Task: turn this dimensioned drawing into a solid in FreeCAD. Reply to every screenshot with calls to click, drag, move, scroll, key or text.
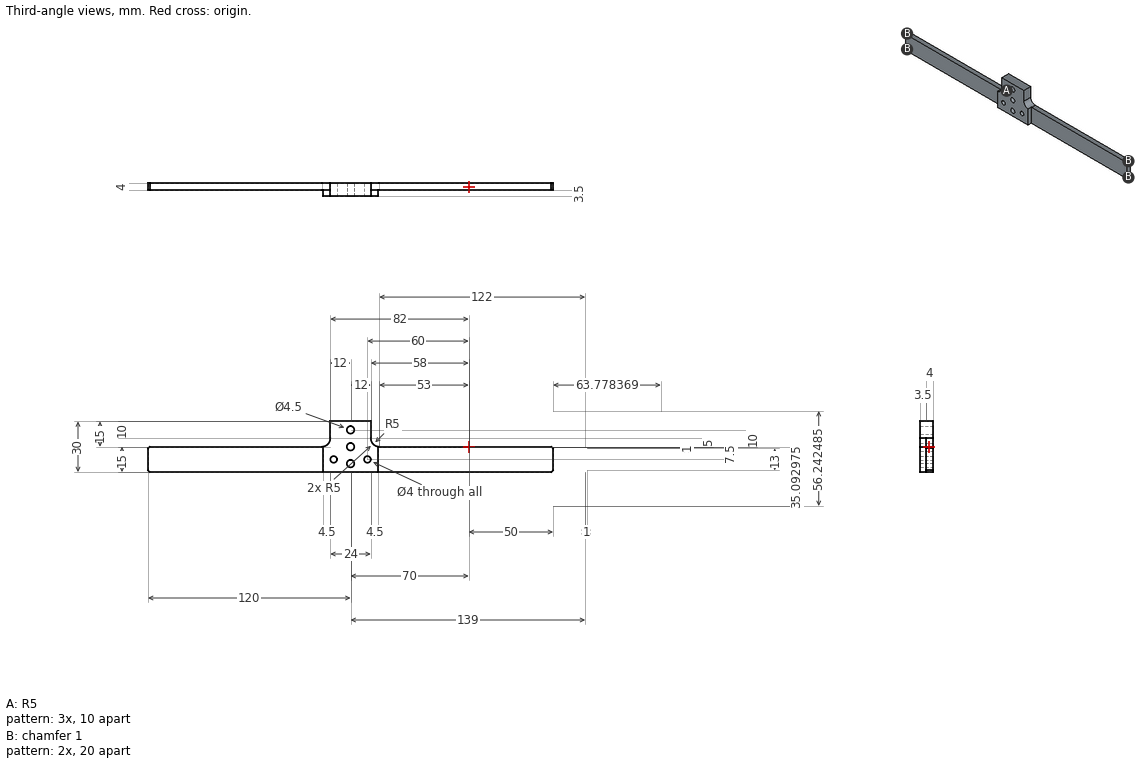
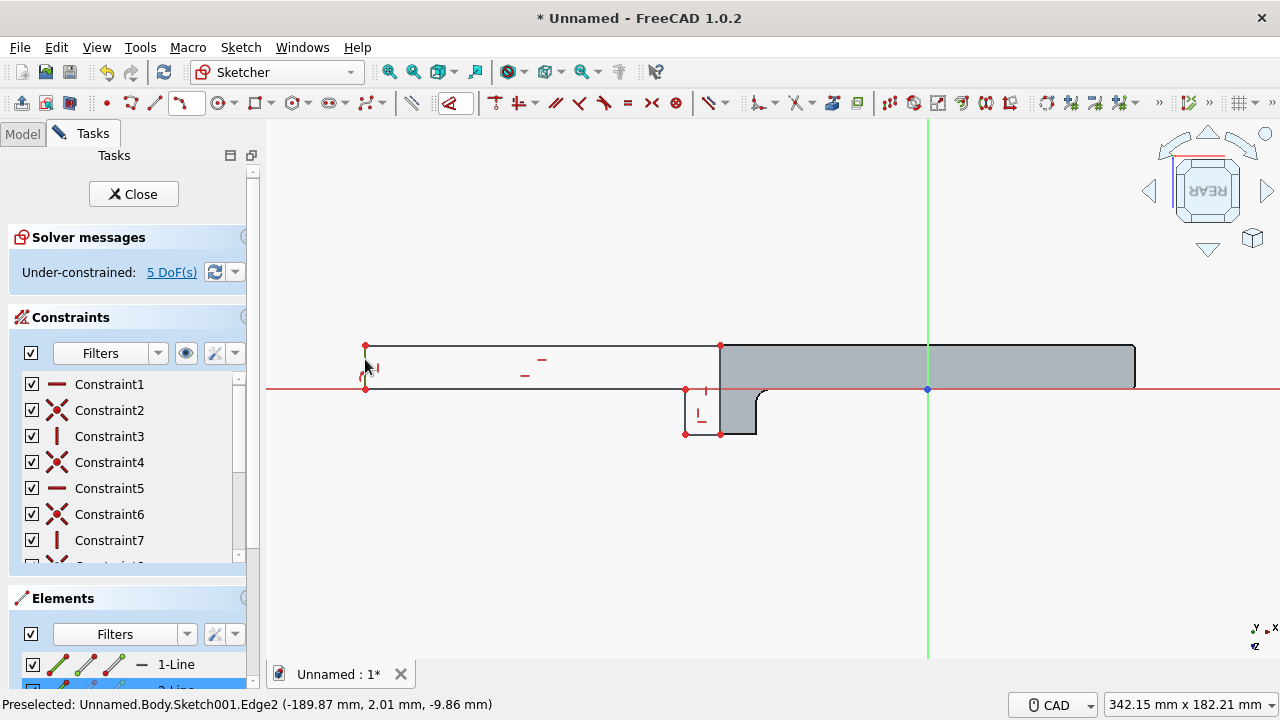
click(468, 104)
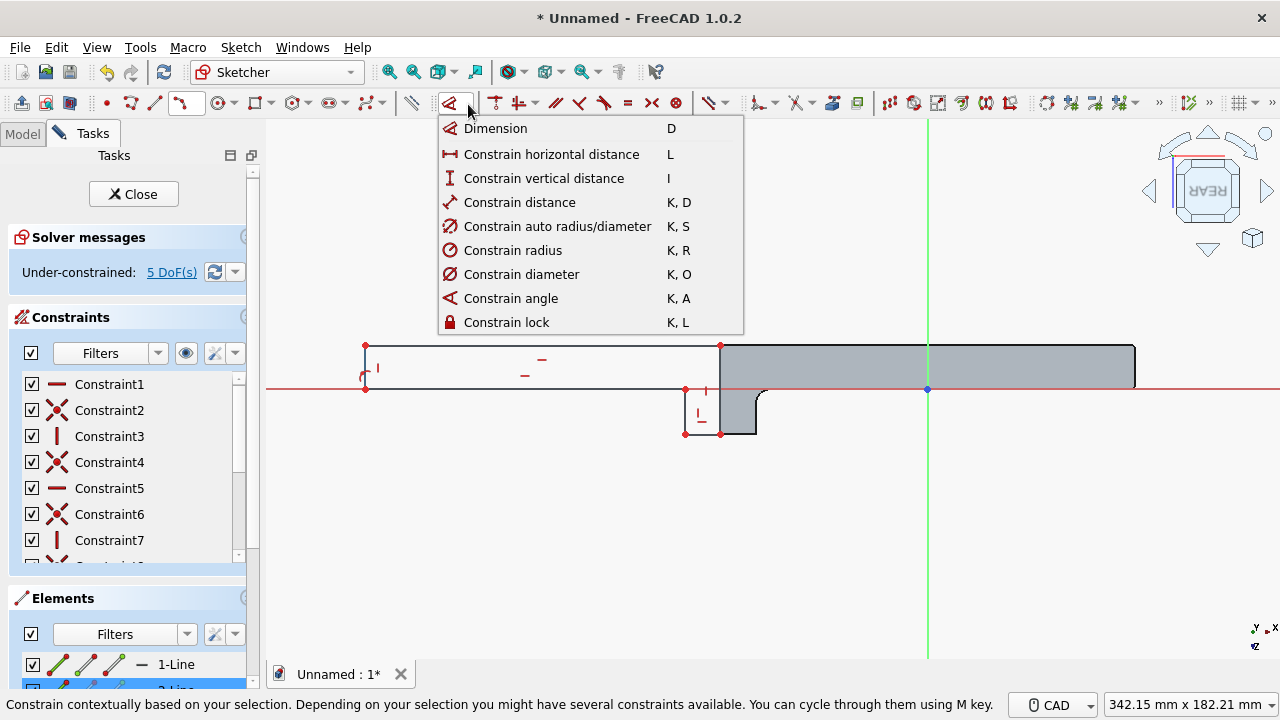
click(591, 178)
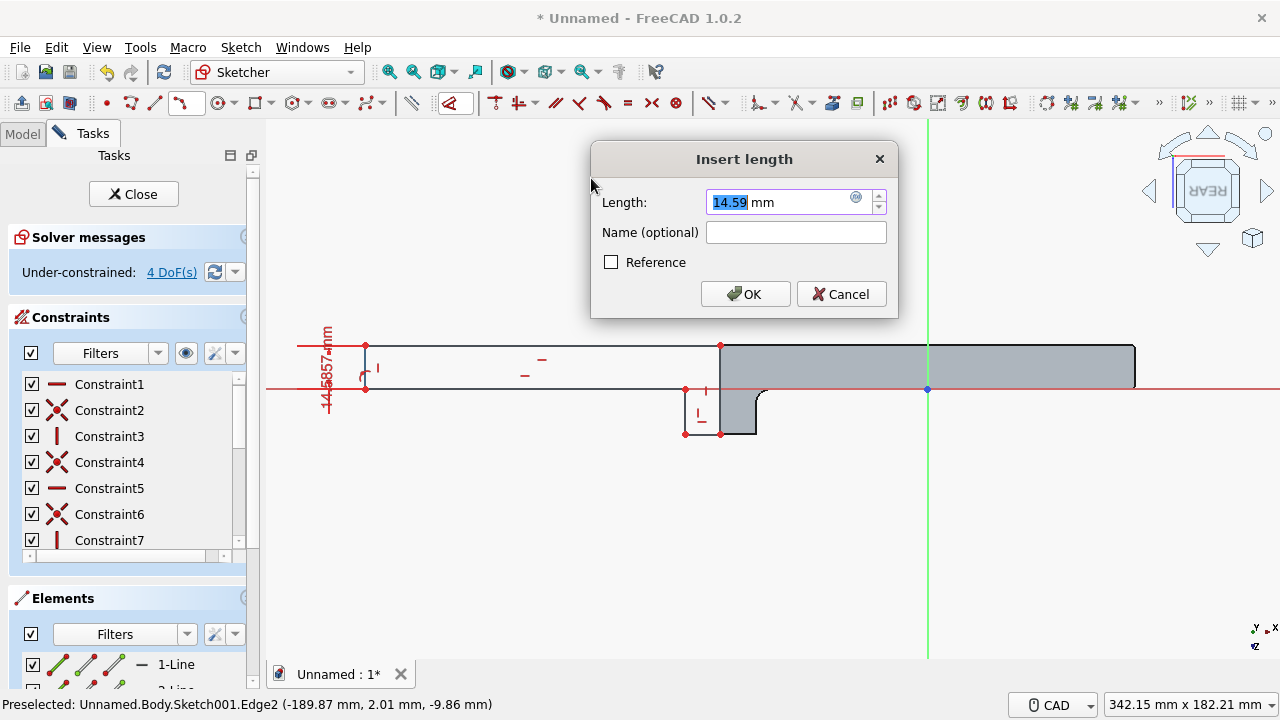
text(15)
key(Return)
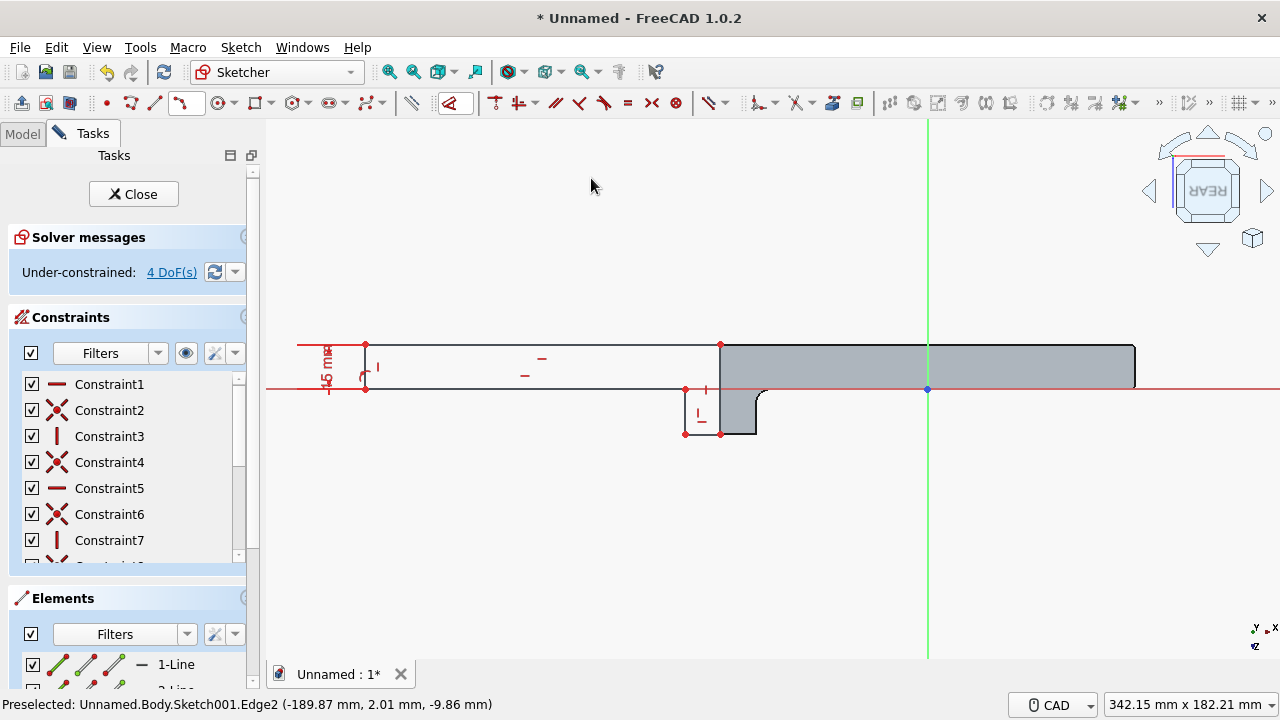
click(685, 403)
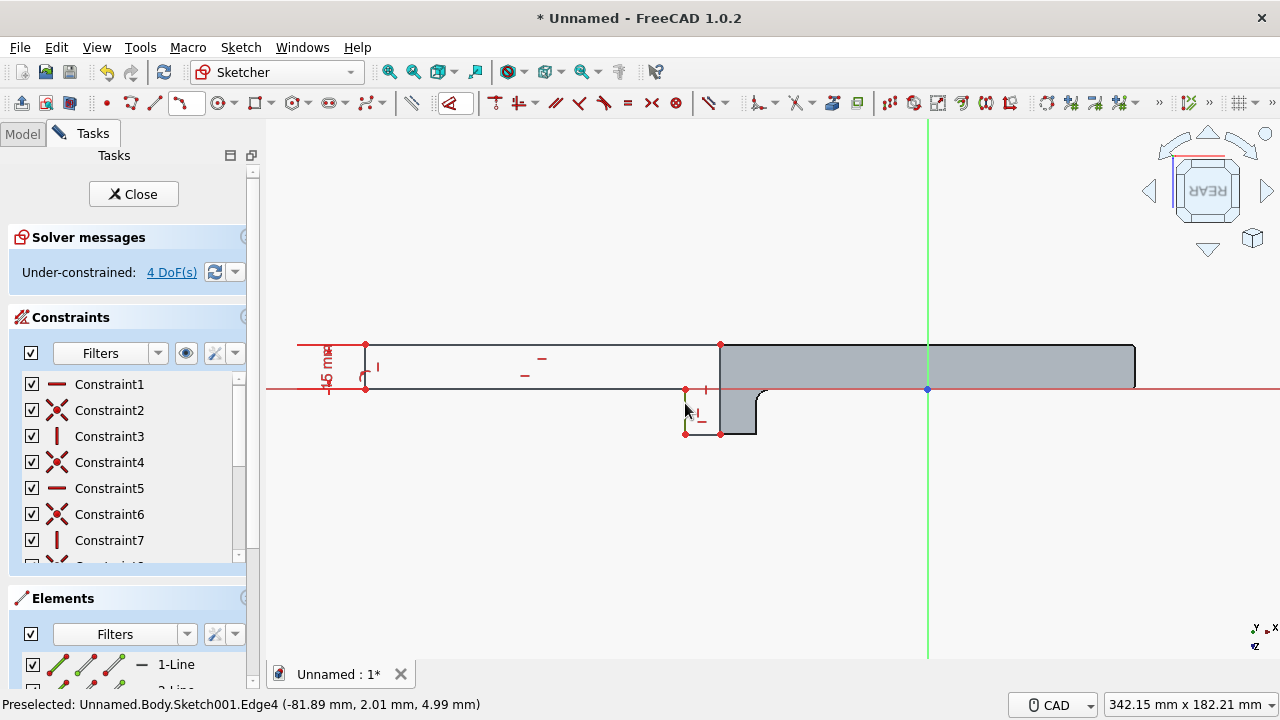
click(468, 104)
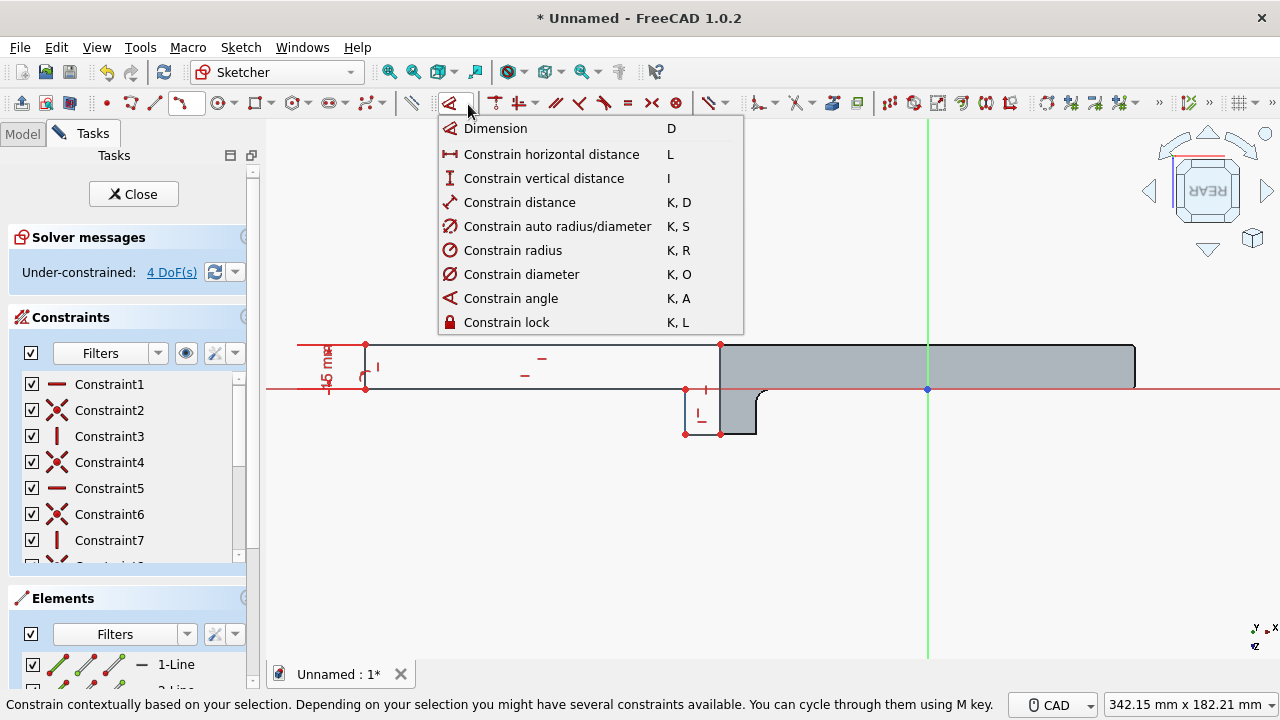
click(591, 178)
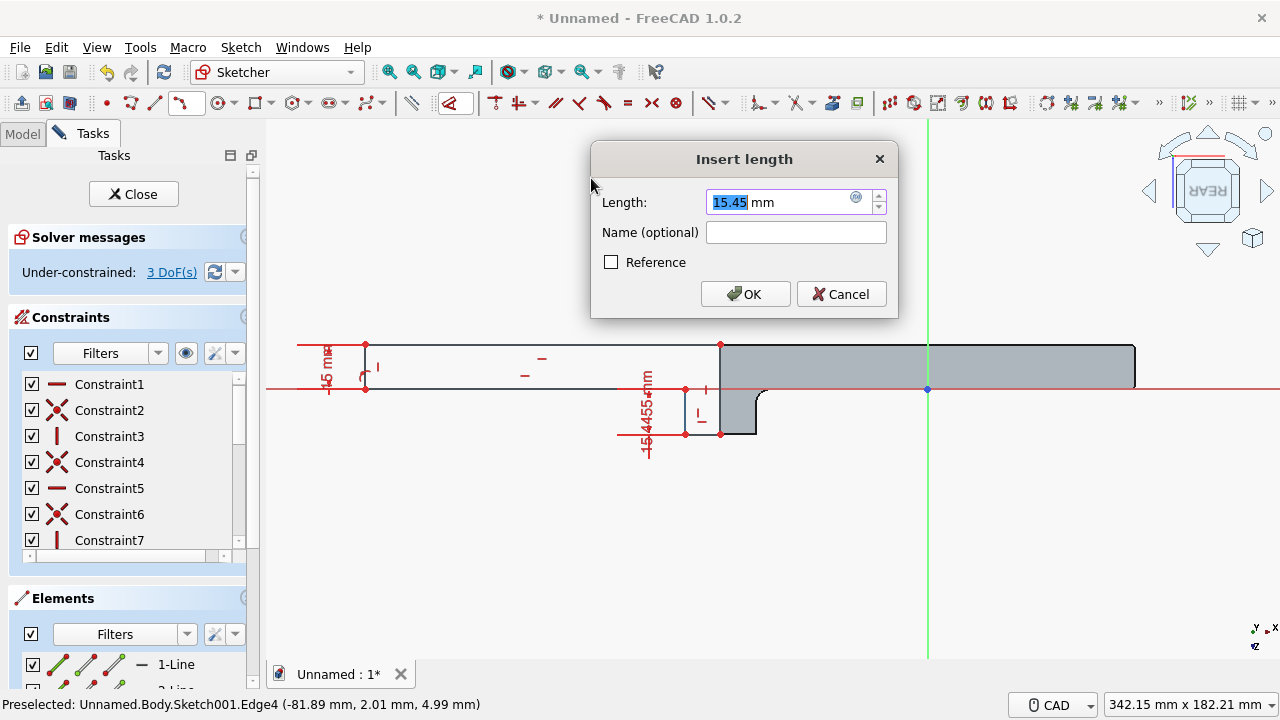
text(15)
key(Return)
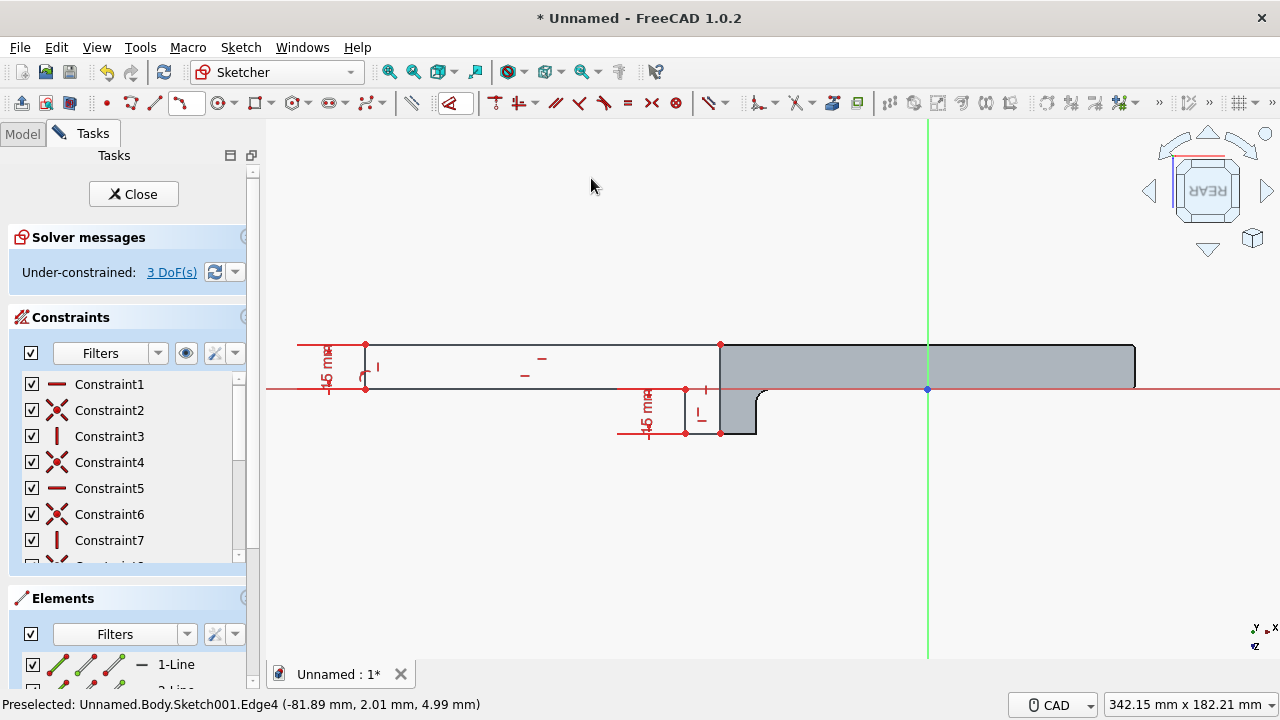
scroll(695, 434, up, 2)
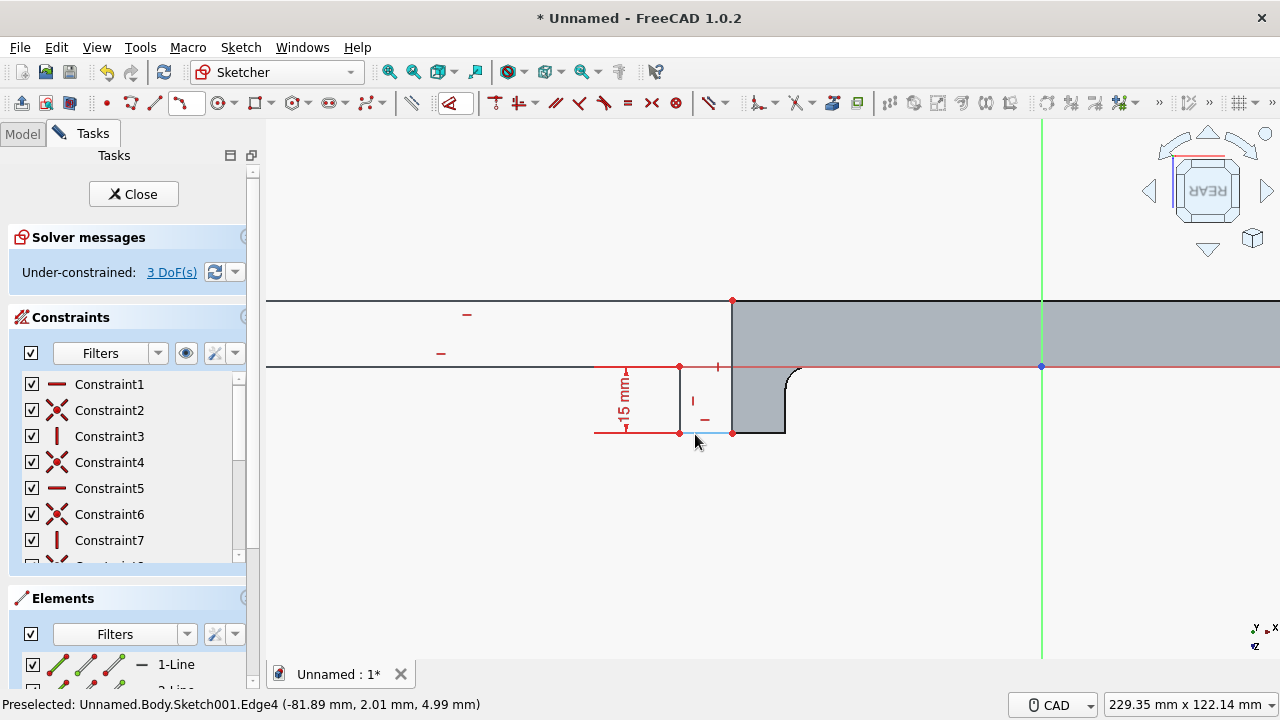
click(696, 433)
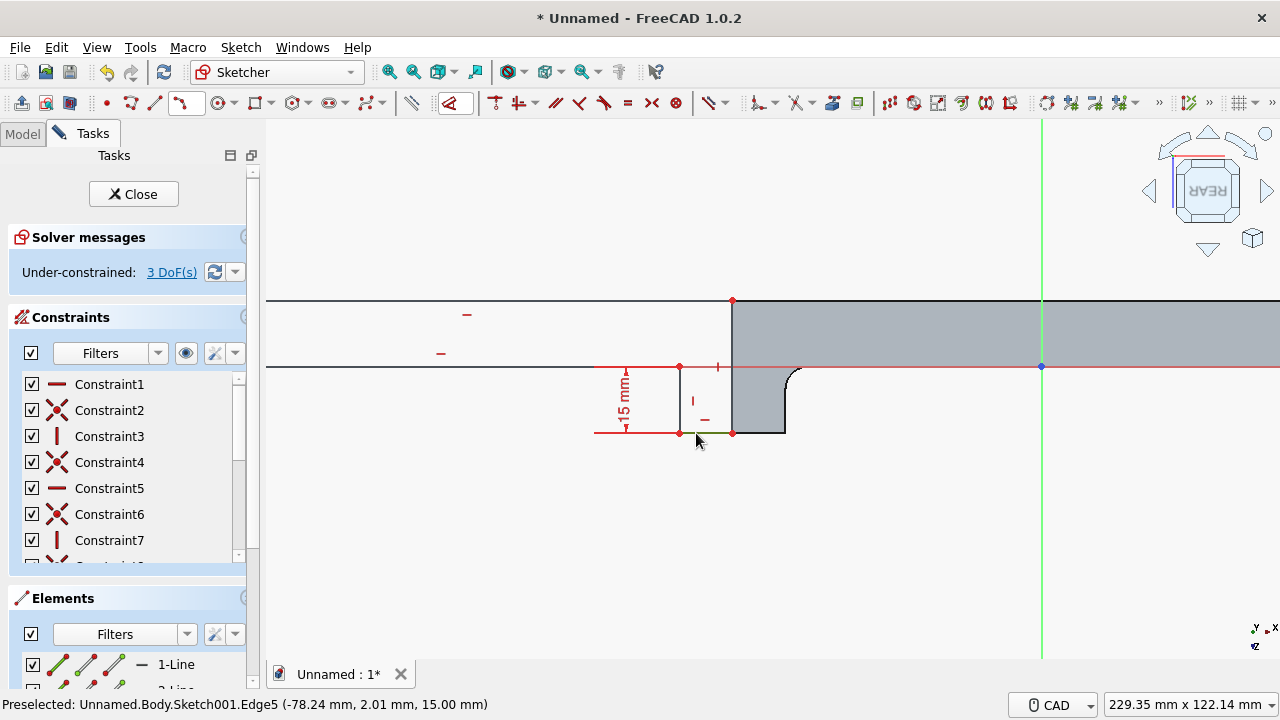
click(468, 104)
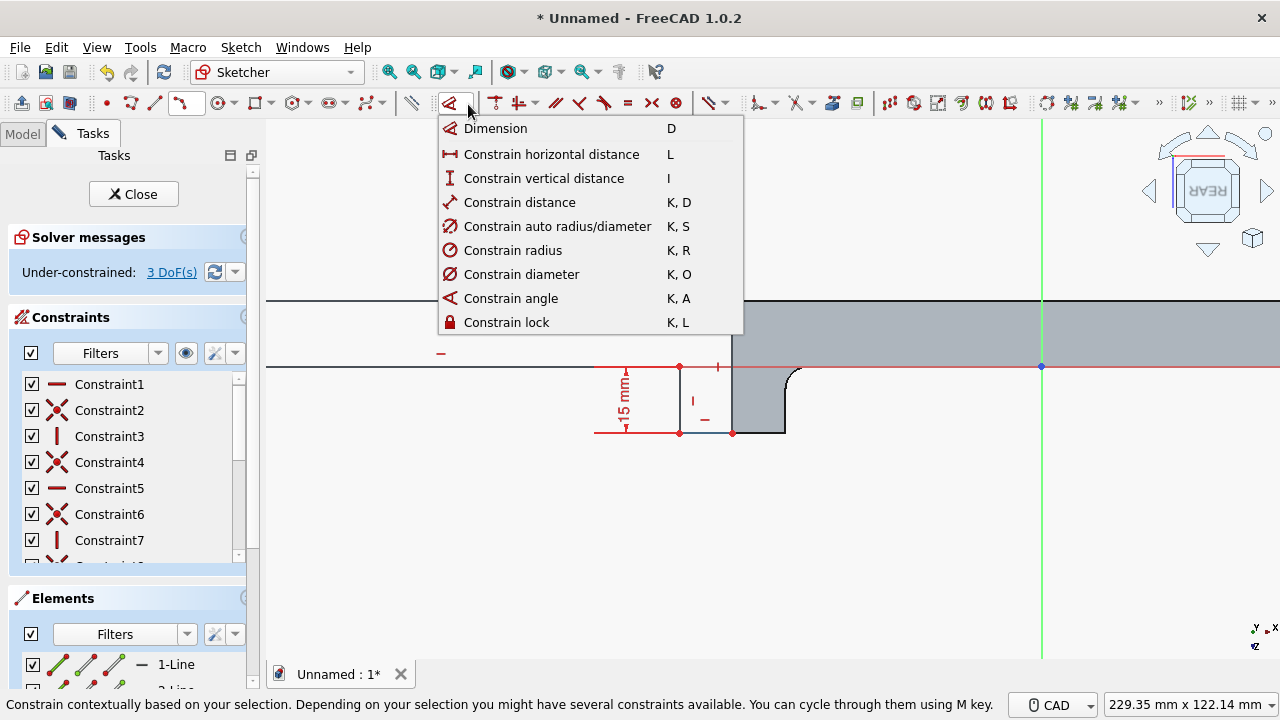
click(591, 154)